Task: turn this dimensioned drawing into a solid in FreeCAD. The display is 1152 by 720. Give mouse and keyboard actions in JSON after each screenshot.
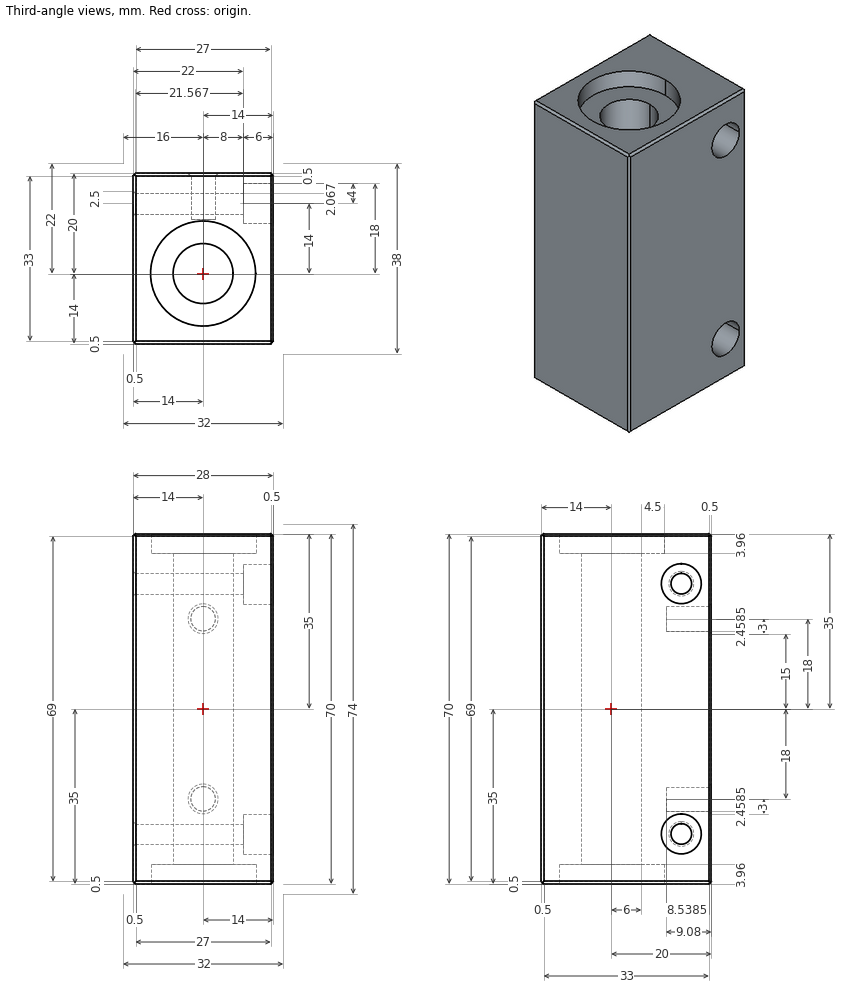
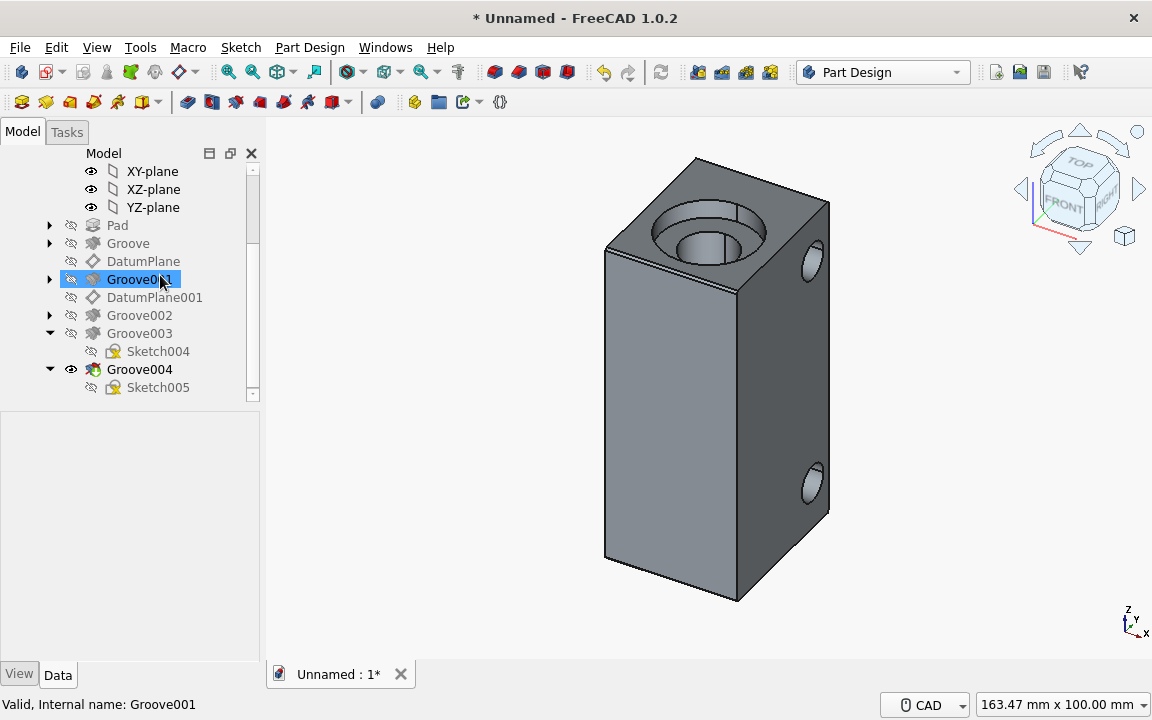
{"action": "scroll", "coordinate": [160, 275], "scroll_direction": "up", "scroll_amount": 15}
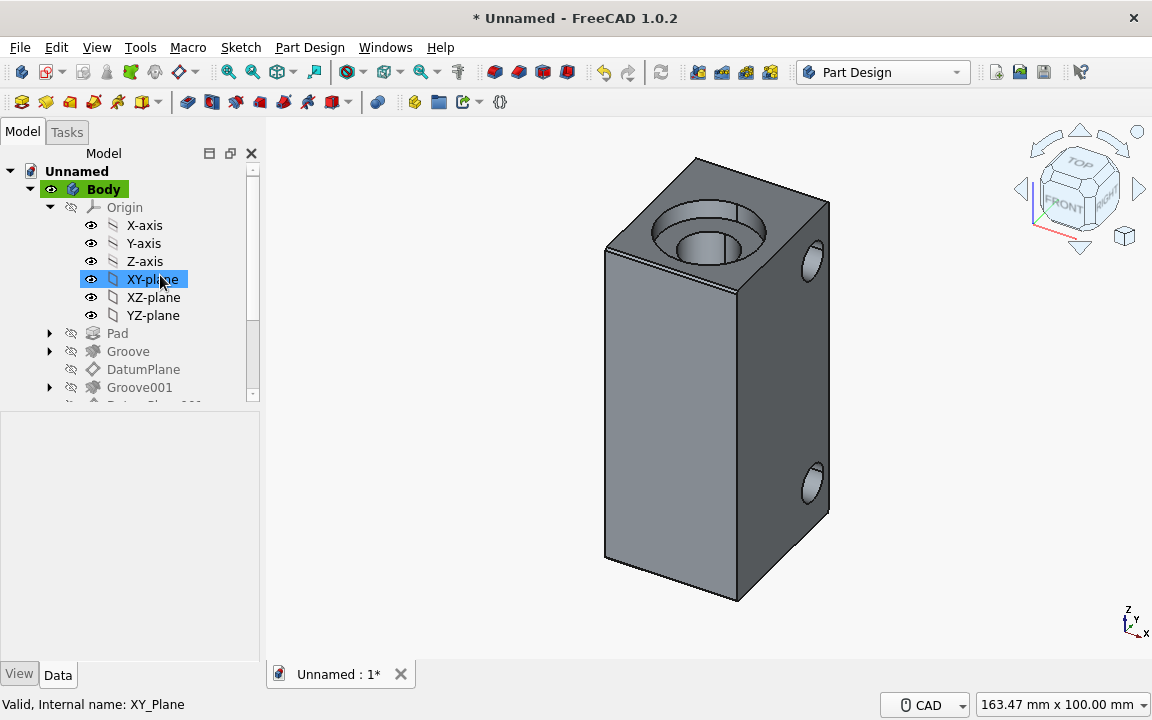
{"action": "left_click", "coordinate": [136, 279]}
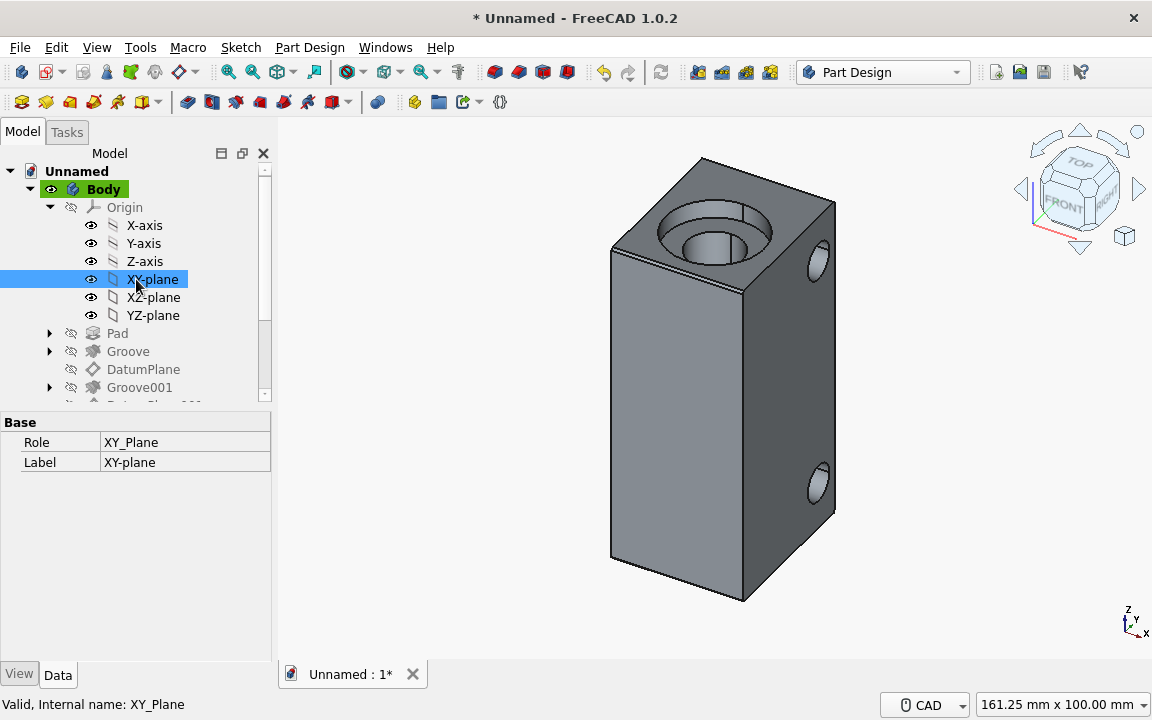
{"action": "left_click", "coordinate": [180, 72]}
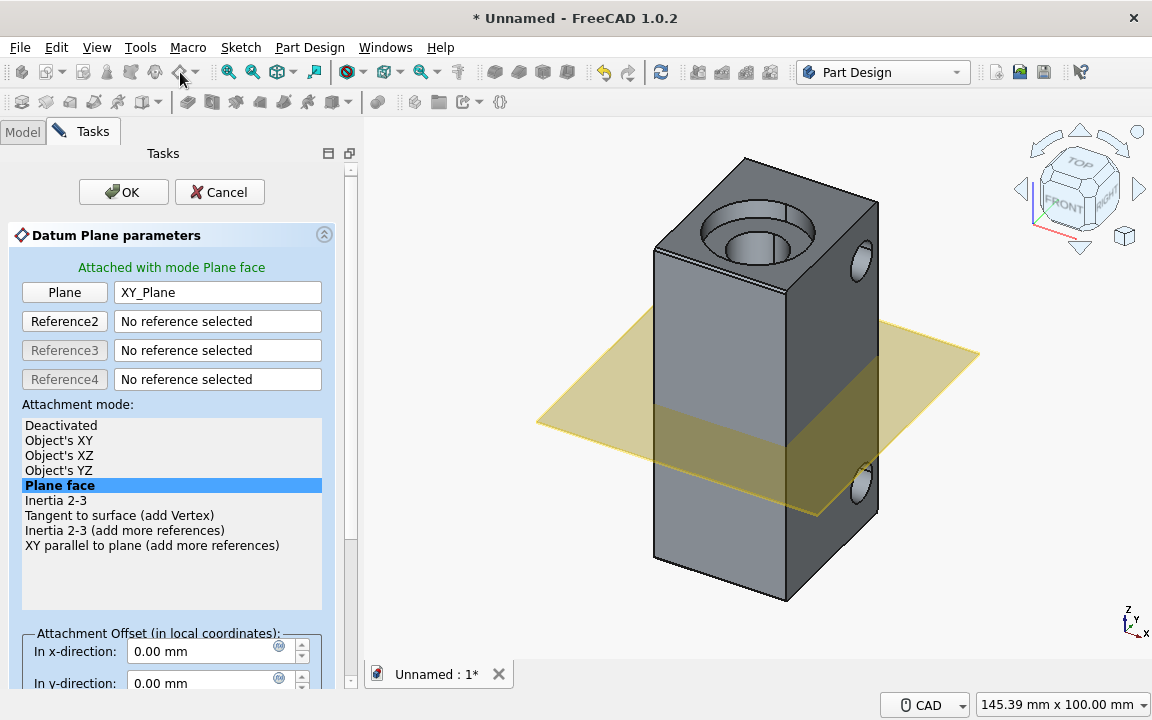
{"action": "scroll", "coordinate": [351, 426], "scroll_direction": "down", "scroll_amount": 2}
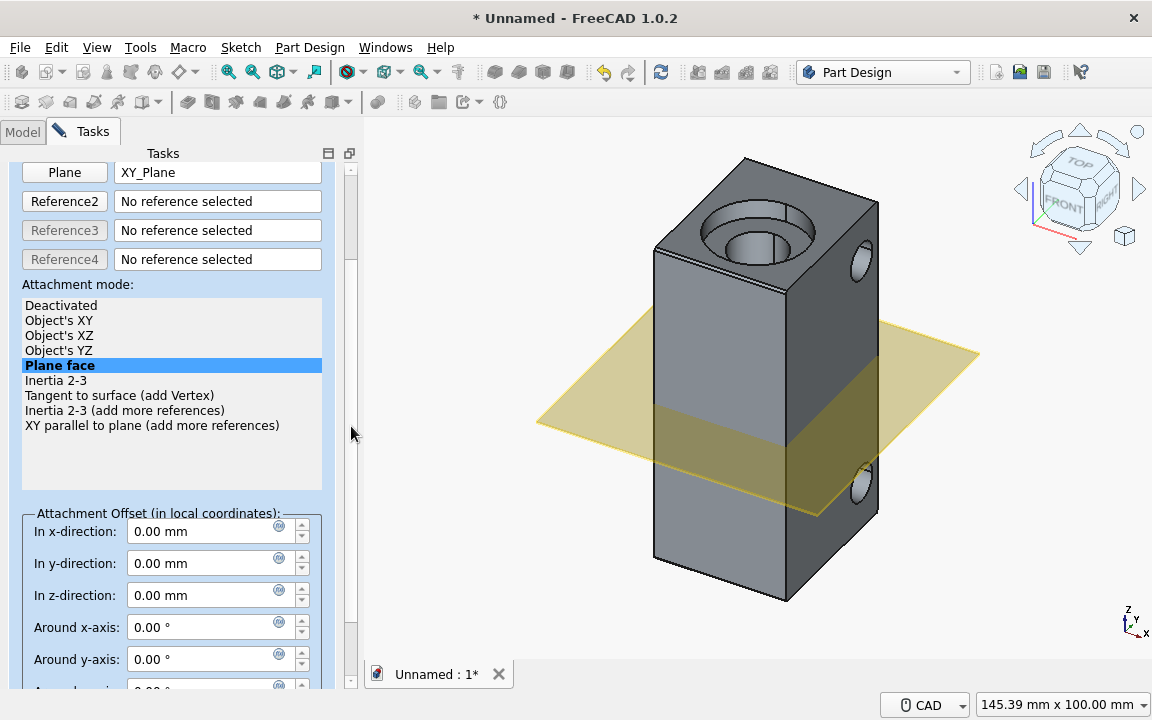
{"action": "triple_click", "coordinate": [210, 595]}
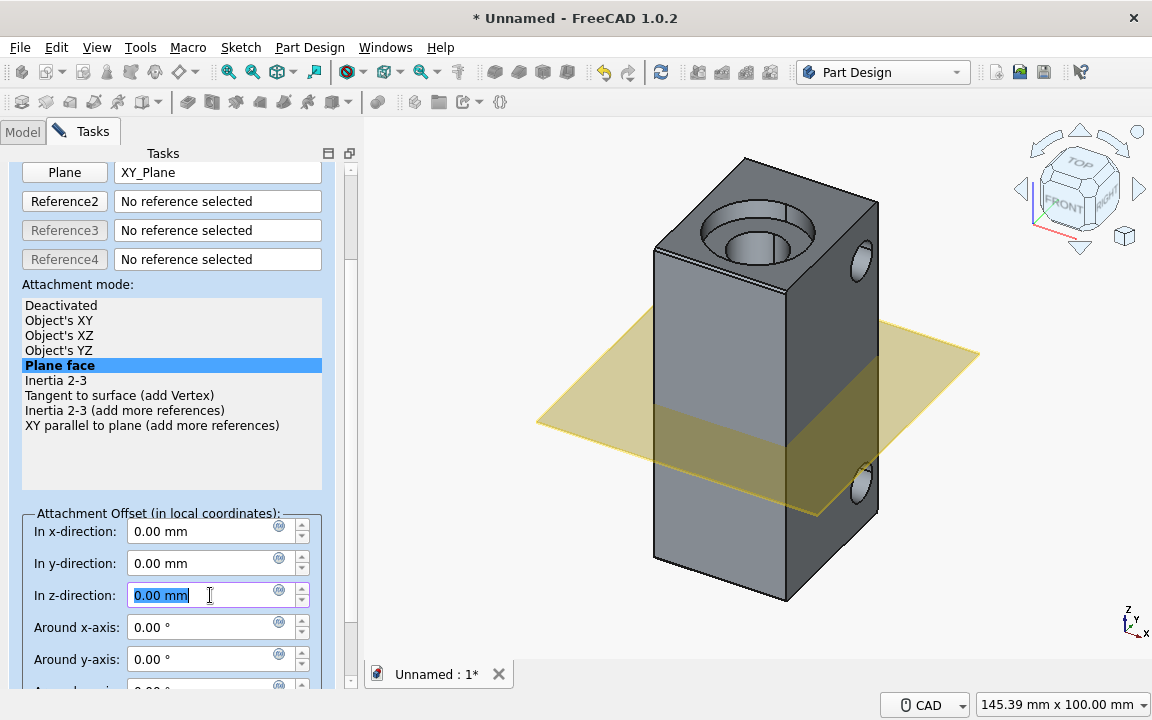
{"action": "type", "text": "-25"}
{"action": "key", "text": "Tab"}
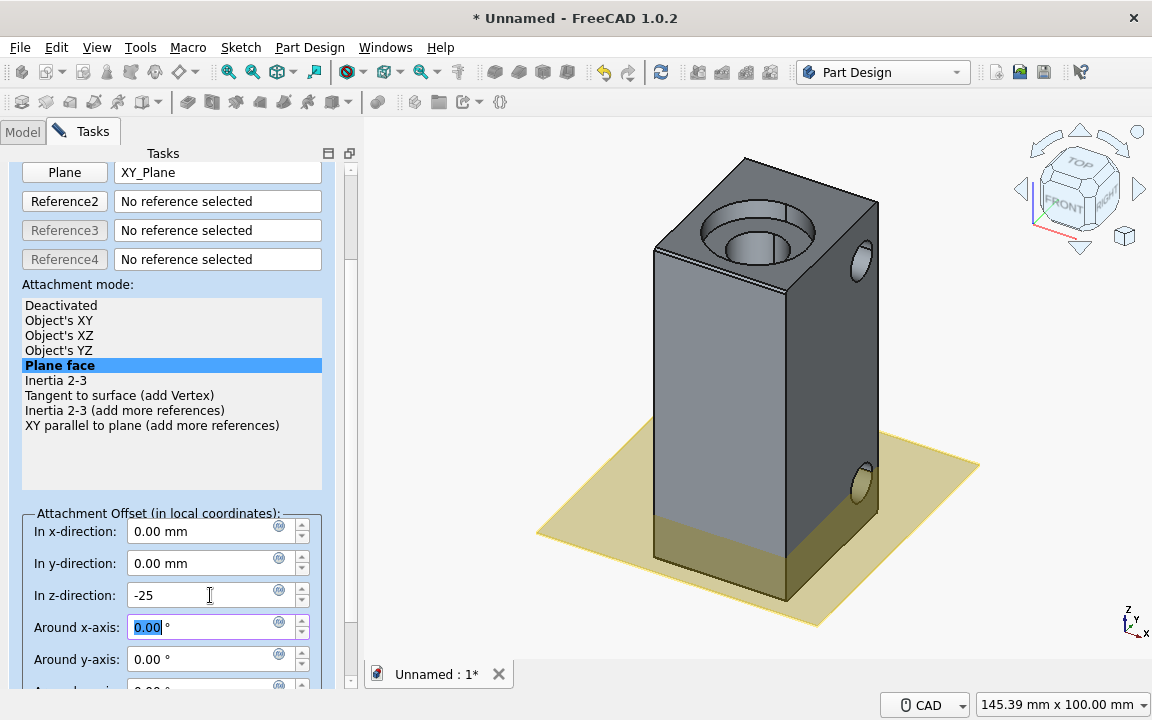
{"action": "scroll", "coordinate": [351, 426], "scroll_direction": "up", "scroll_amount": 3}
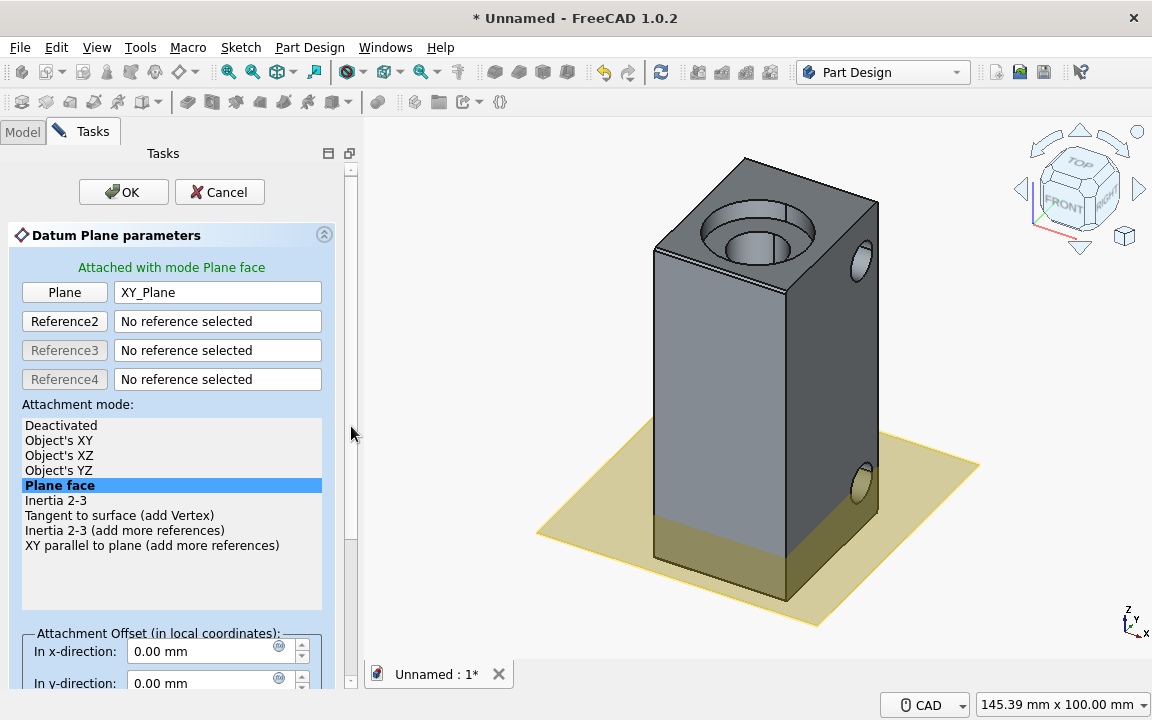
{"action": "left_click", "coordinate": [124, 192]}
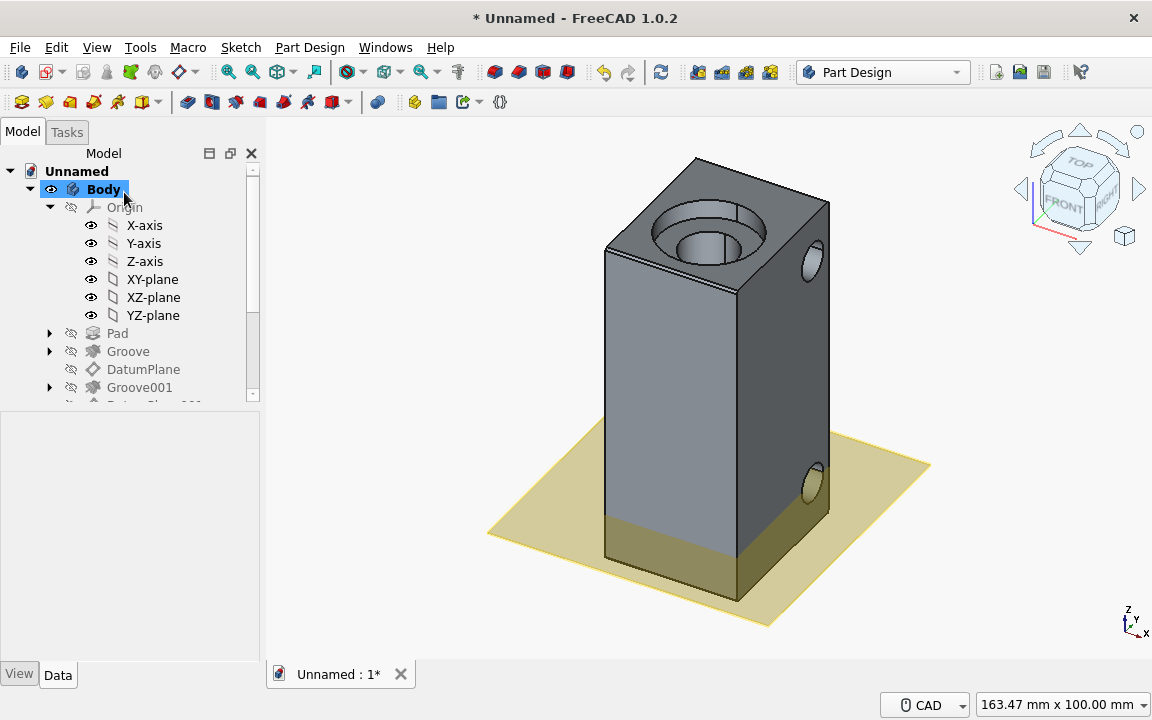
{"action": "scroll", "coordinate": [100, 275], "scroll_direction": "down", "scroll_amount": 3}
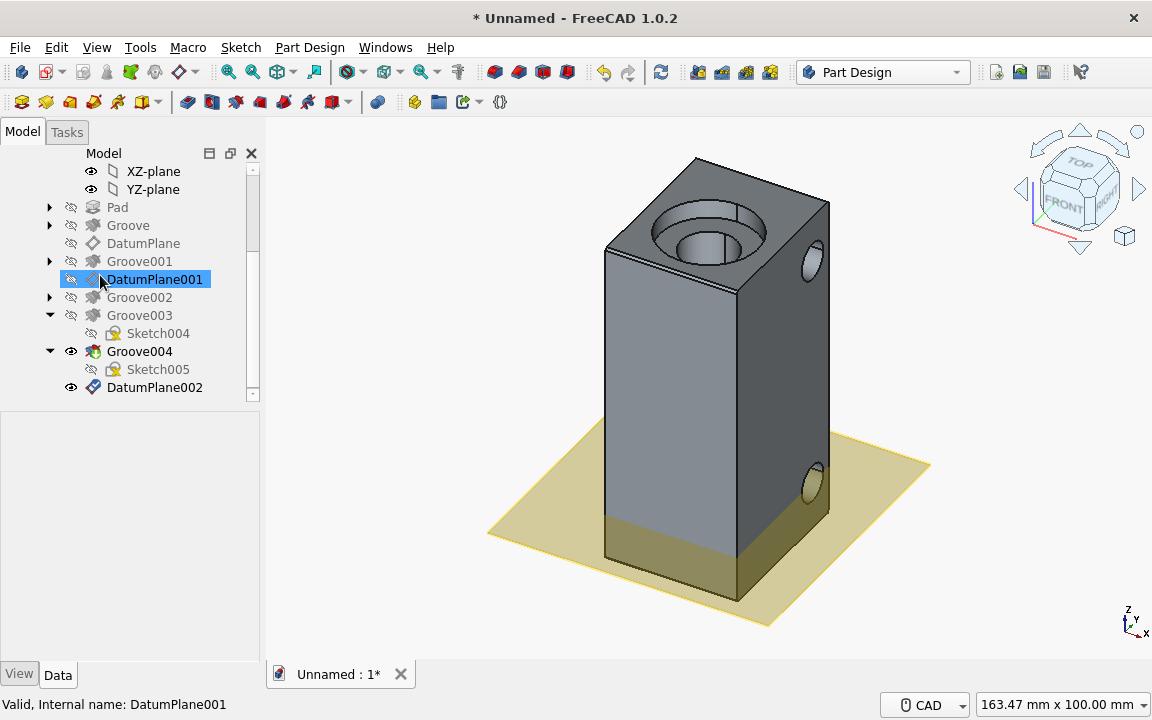
{"action": "left_click", "coordinate": [116, 387]}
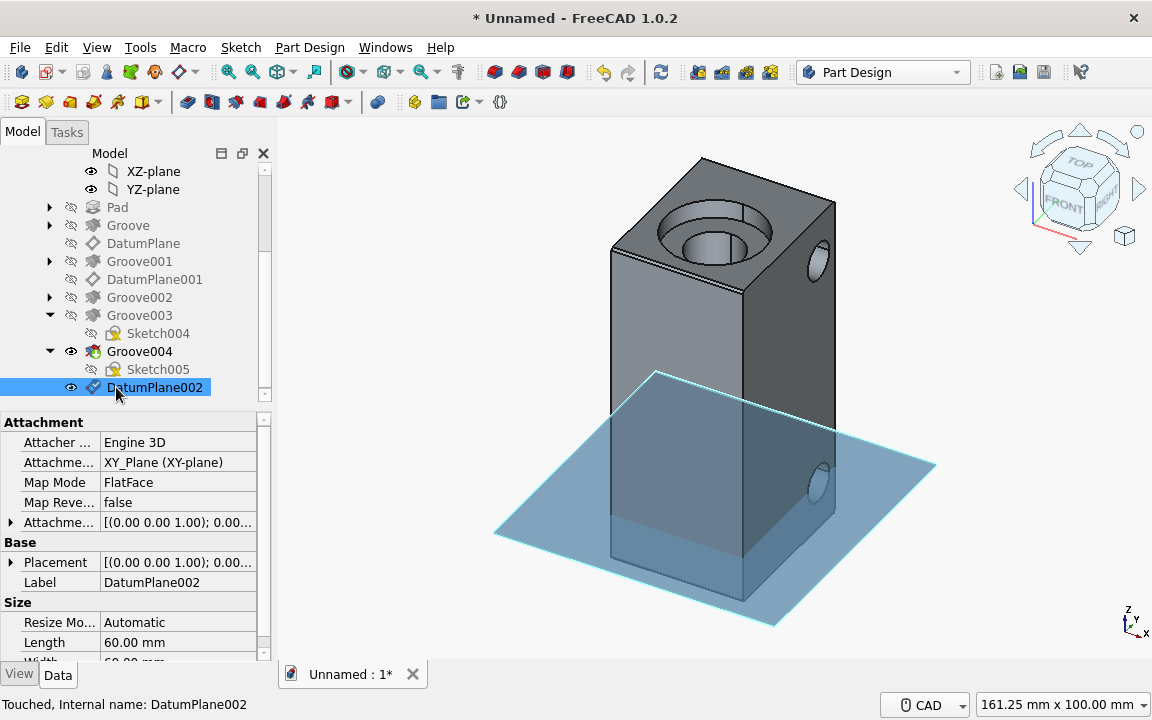
{"action": "left_click", "coordinate": [46, 72]}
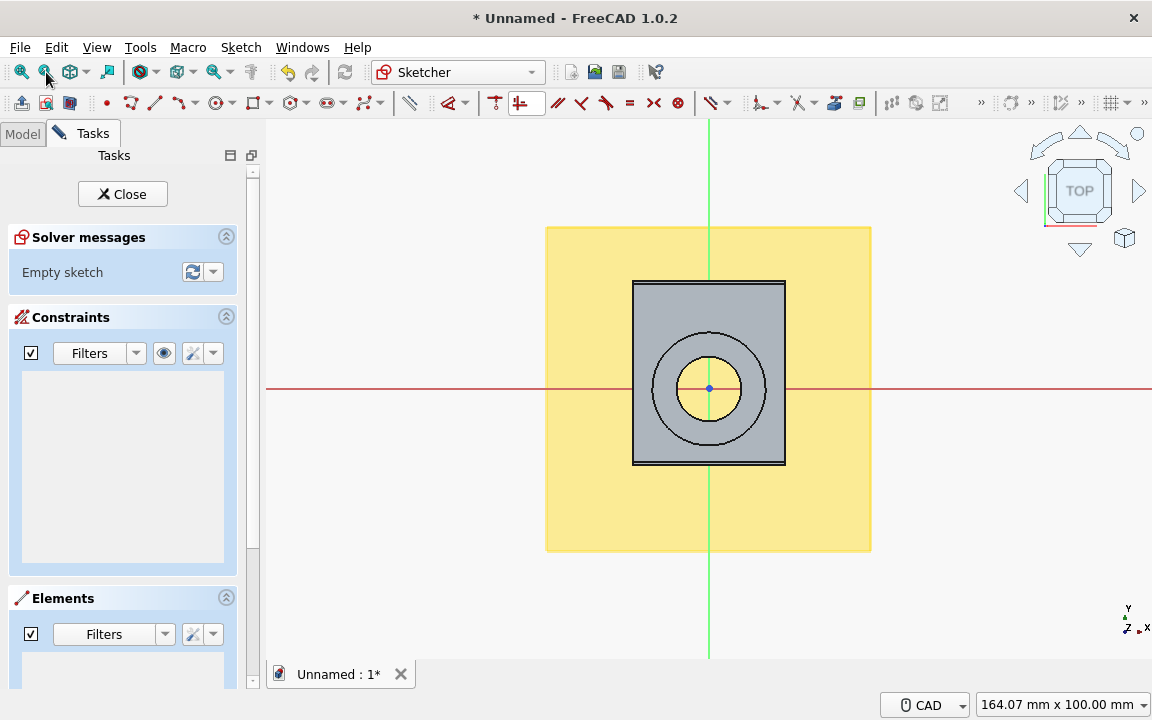
{"action": "left_click", "coordinate": [70, 104]}